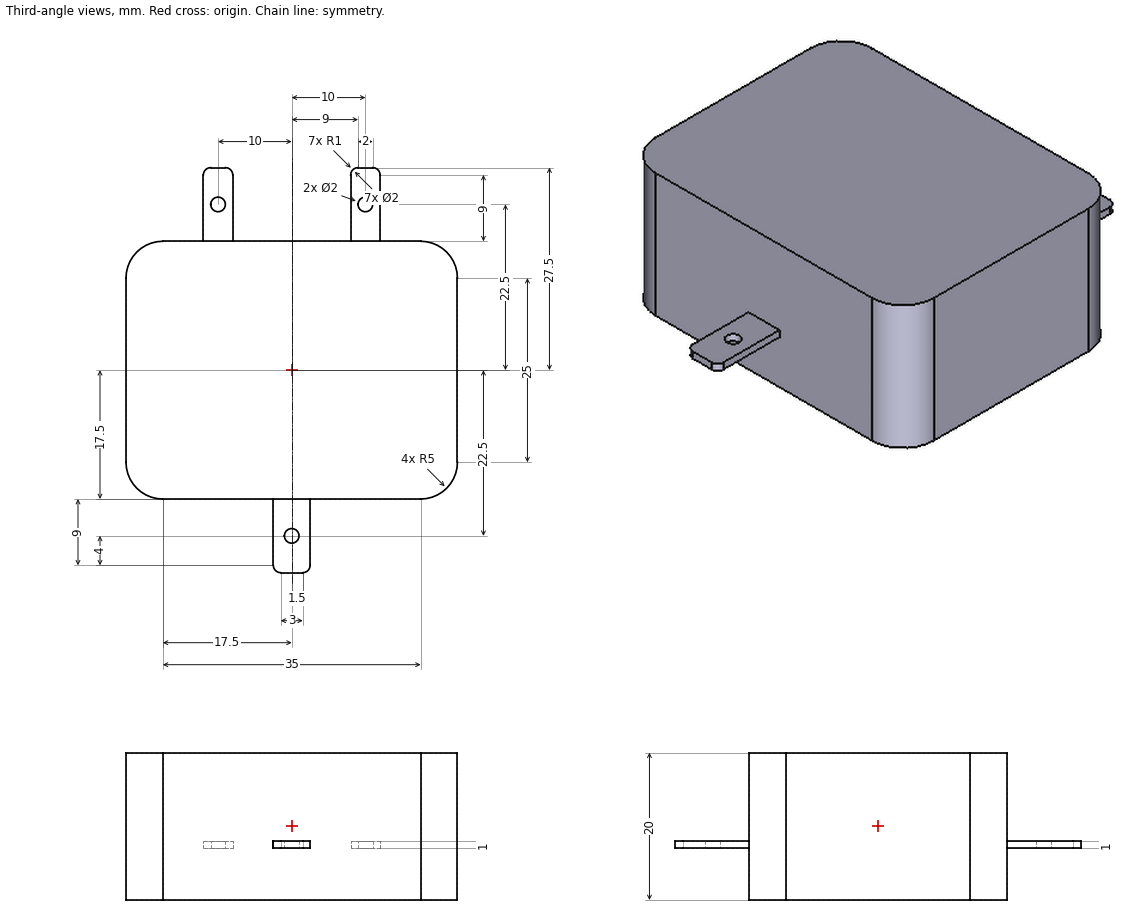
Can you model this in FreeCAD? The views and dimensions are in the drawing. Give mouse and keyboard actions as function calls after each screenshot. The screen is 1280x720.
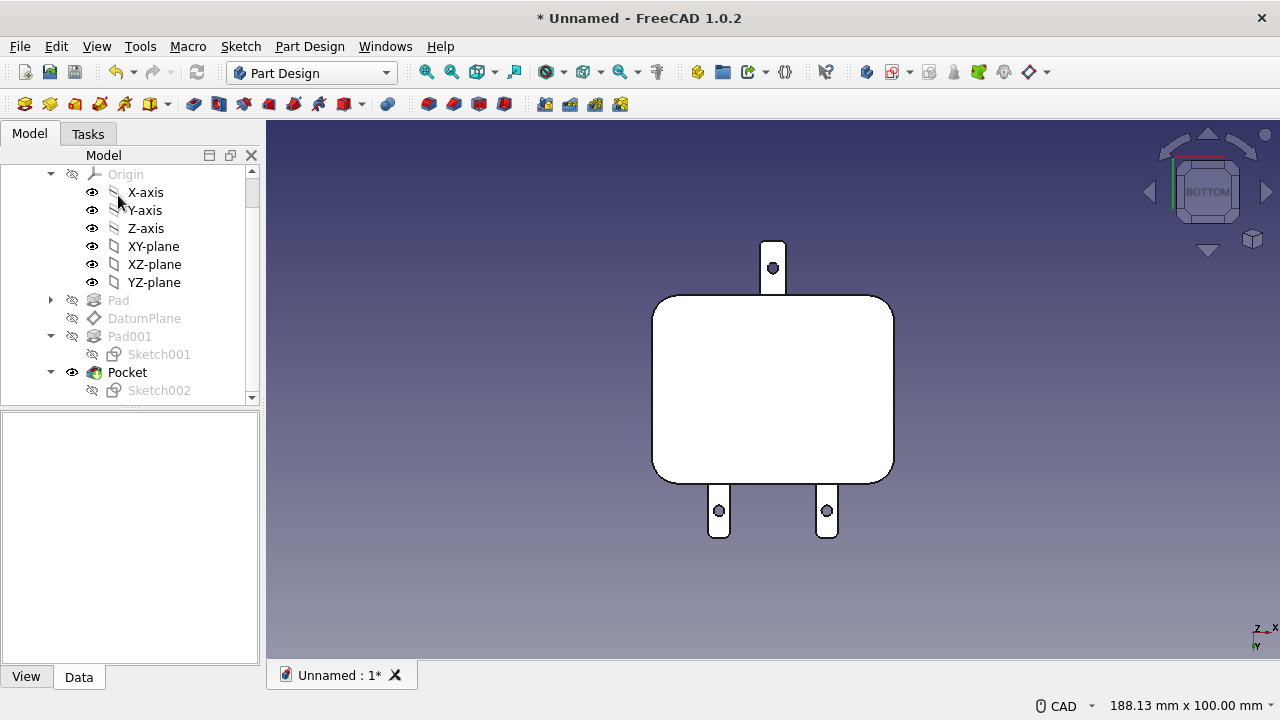
key(0)